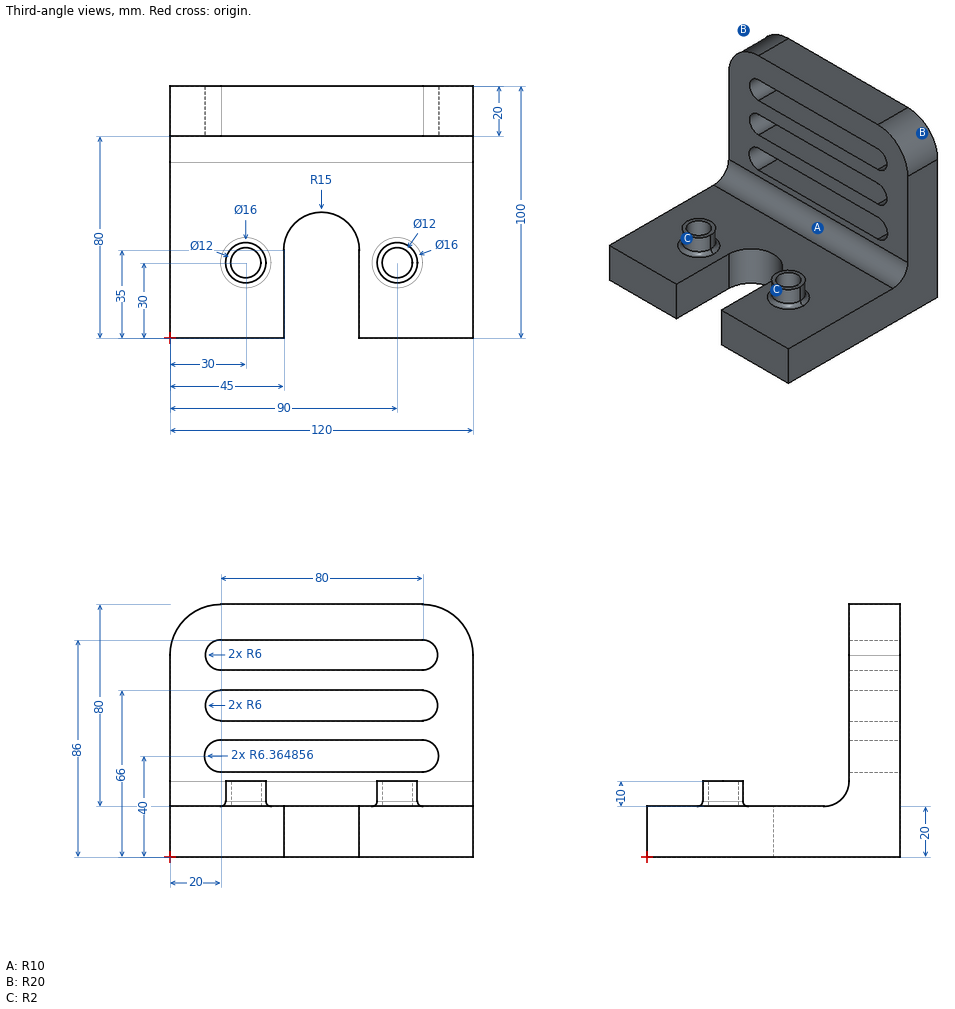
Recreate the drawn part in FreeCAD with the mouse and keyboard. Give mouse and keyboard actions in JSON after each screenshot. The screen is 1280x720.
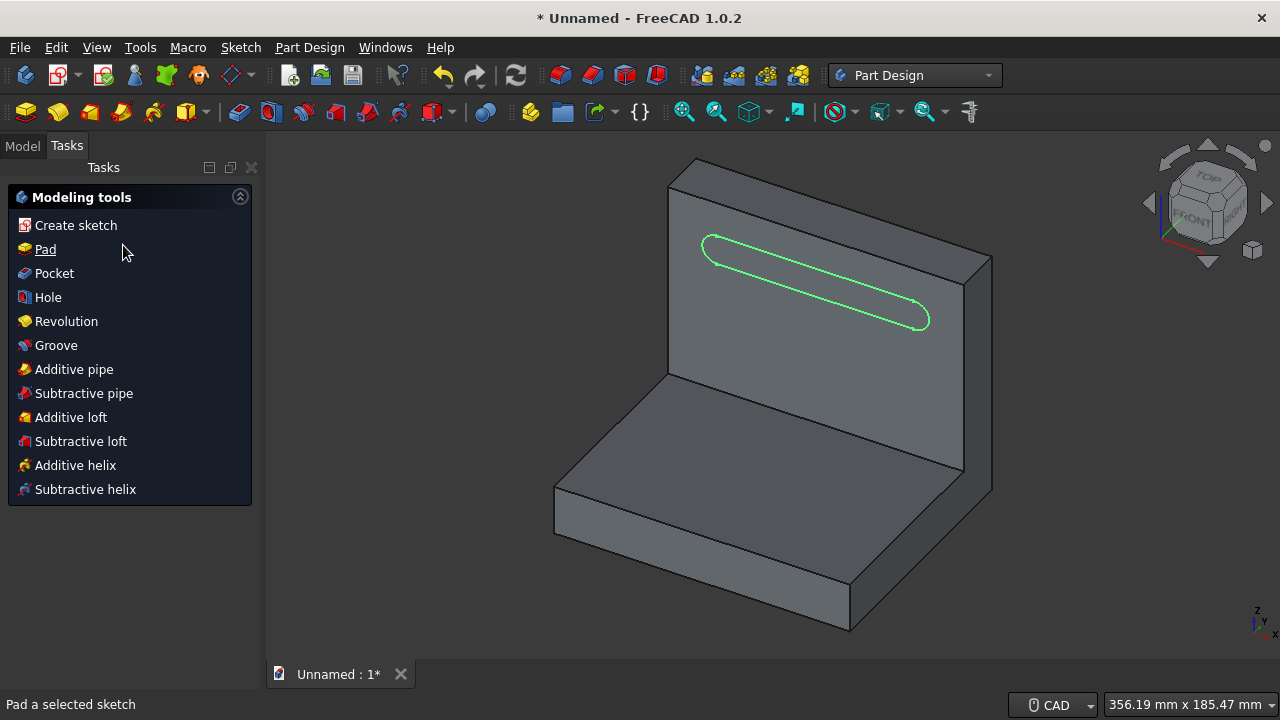
{"action": "left_click", "coordinate": [240, 112]}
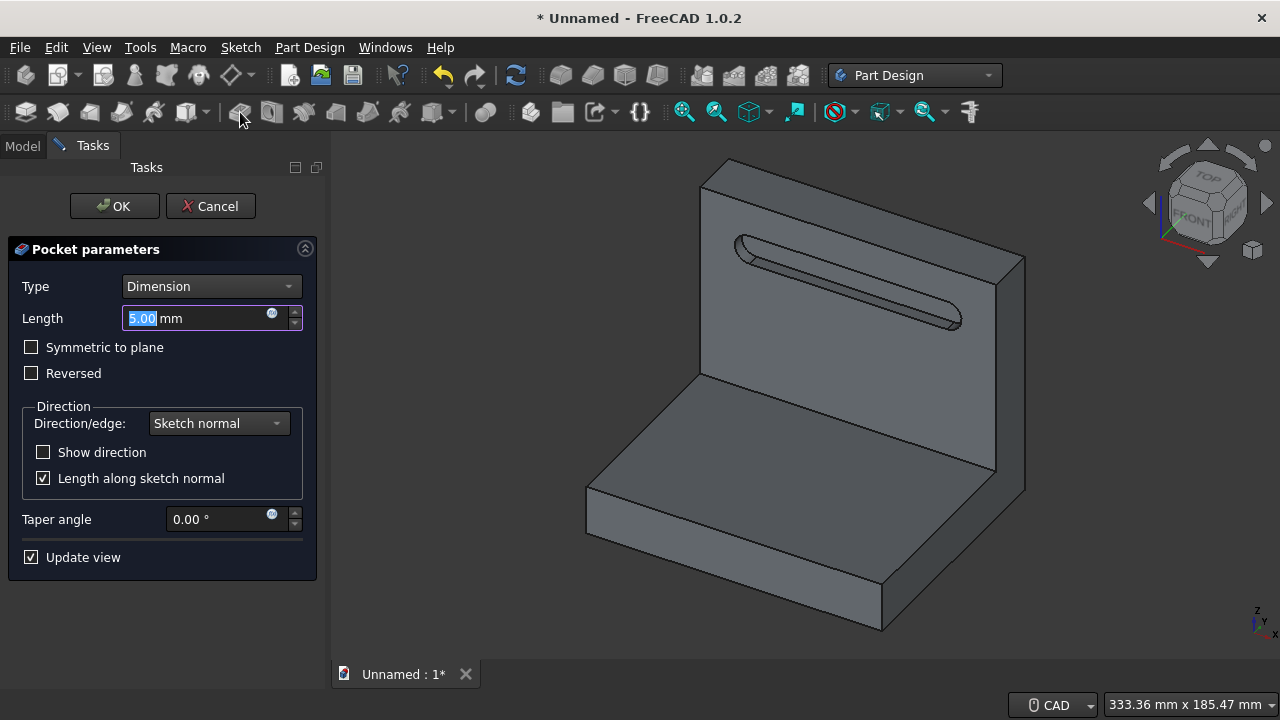
{"action": "left_click", "coordinate": [212, 286]}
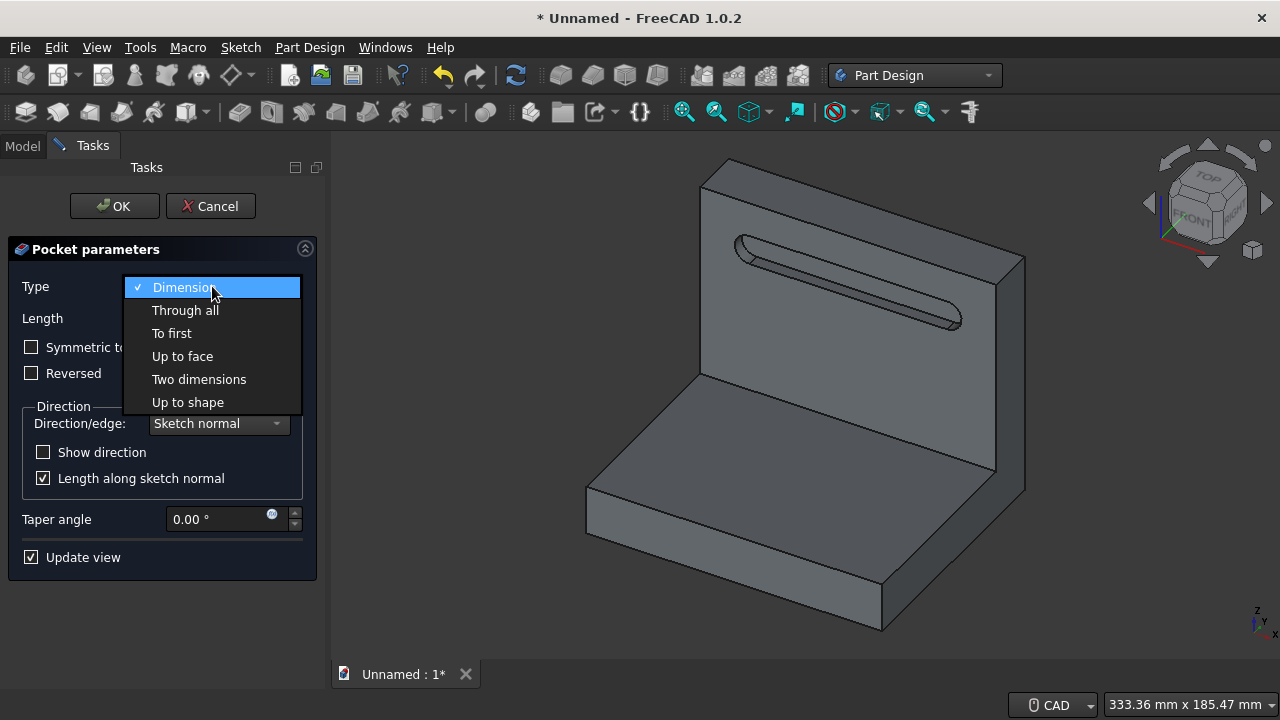
{"action": "left_click", "coordinate": [212, 310]}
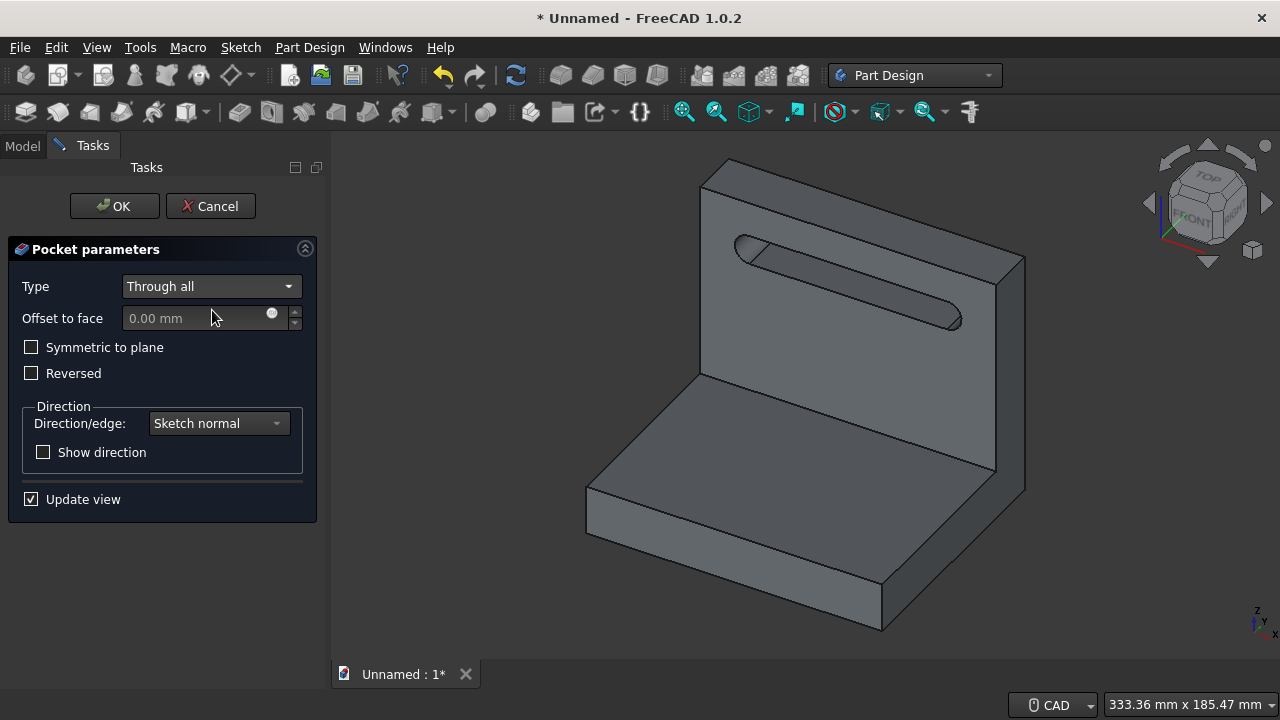
{"action": "left_click", "coordinate": [115, 206]}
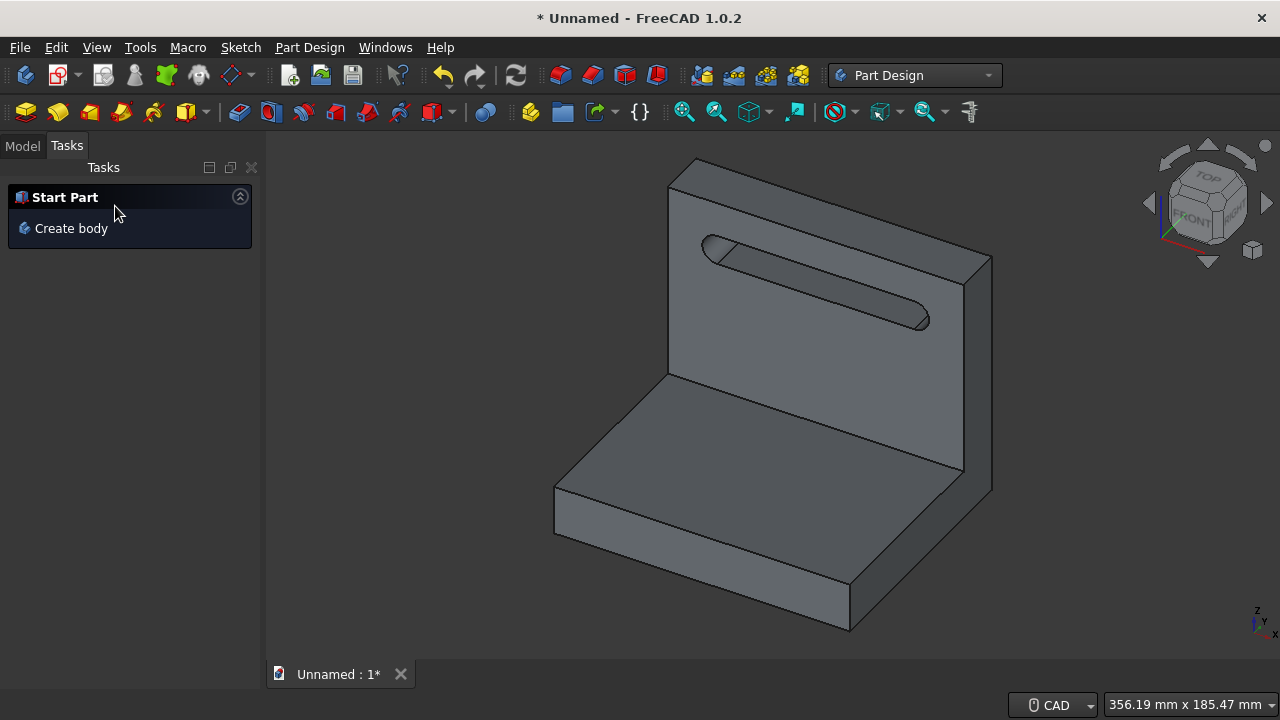
{"action": "left_click", "coordinate": [900, 383]}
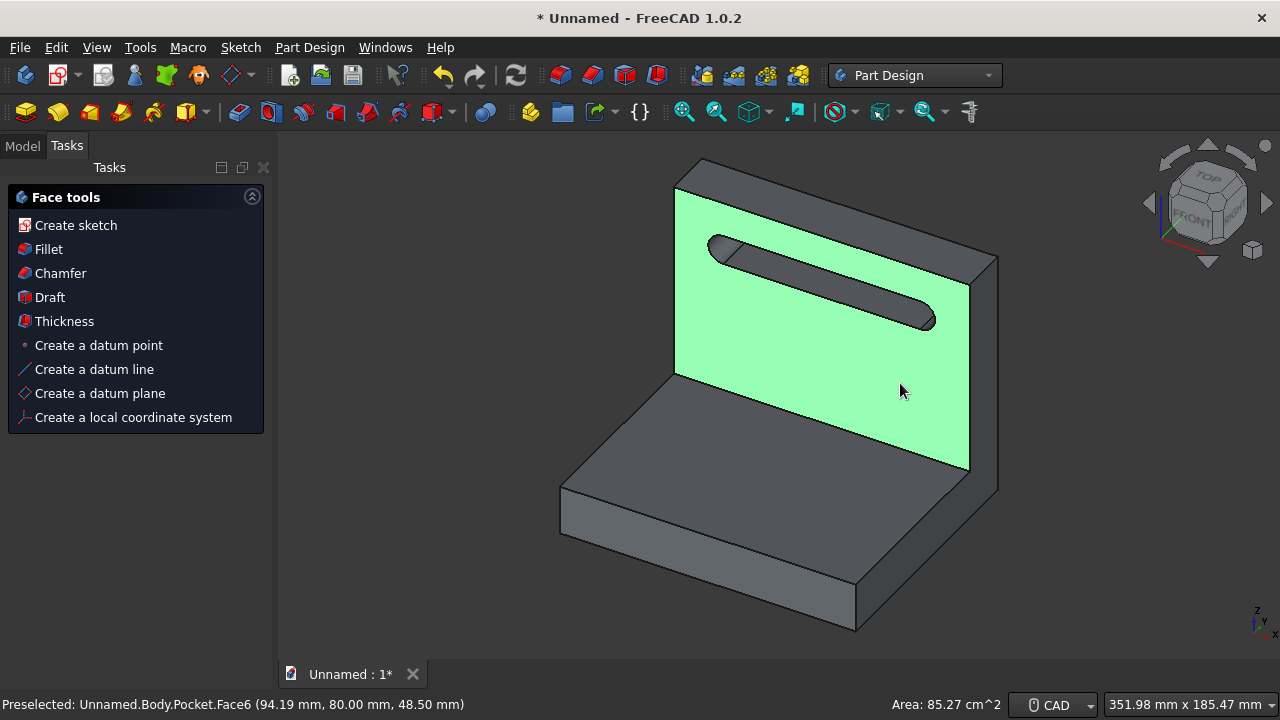
{"action": "left_click", "coordinate": [58, 76]}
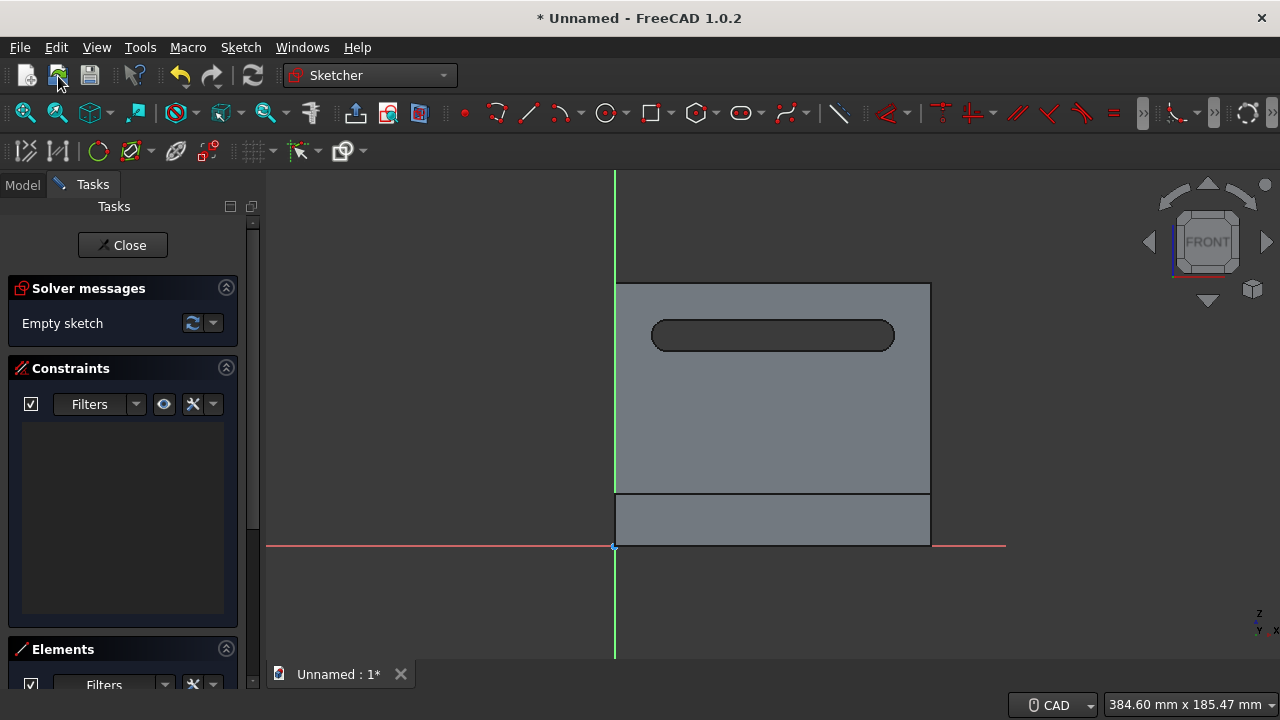
{"action": "key", "text": "q s"}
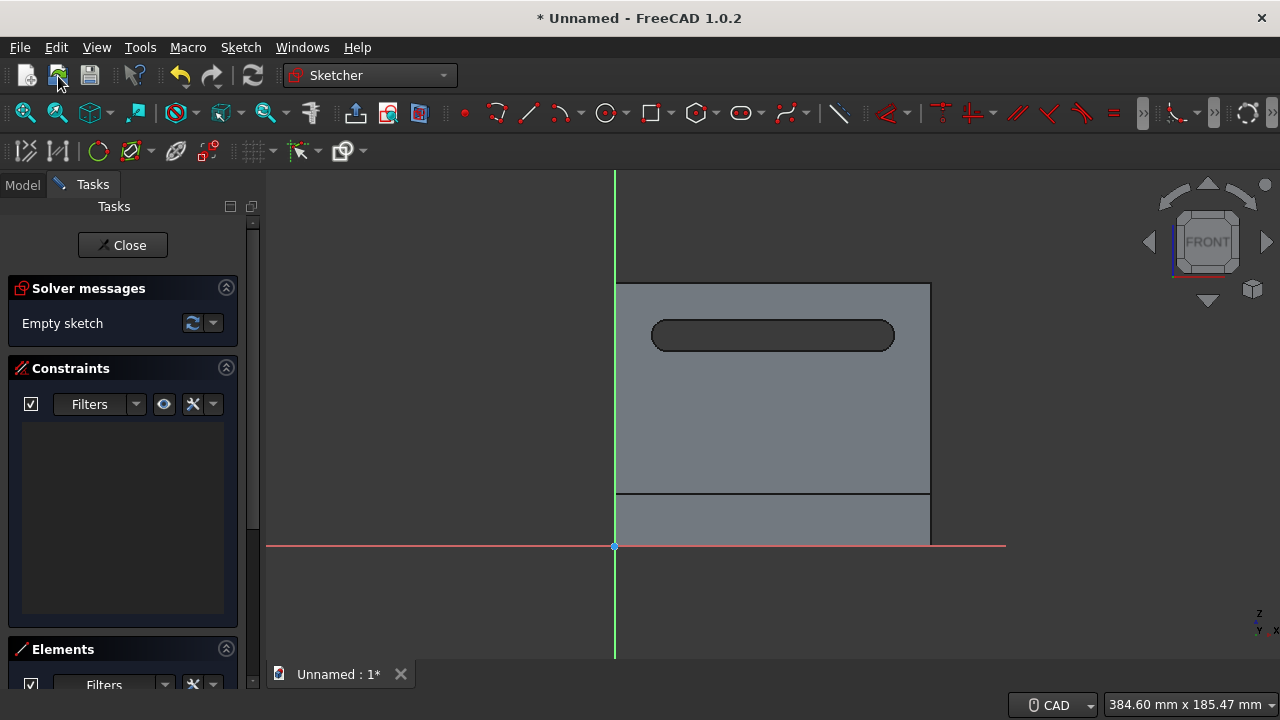
{"action": "scroll", "coordinate": [815, 514], "scroll_direction": "up", "scroll_amount": 3}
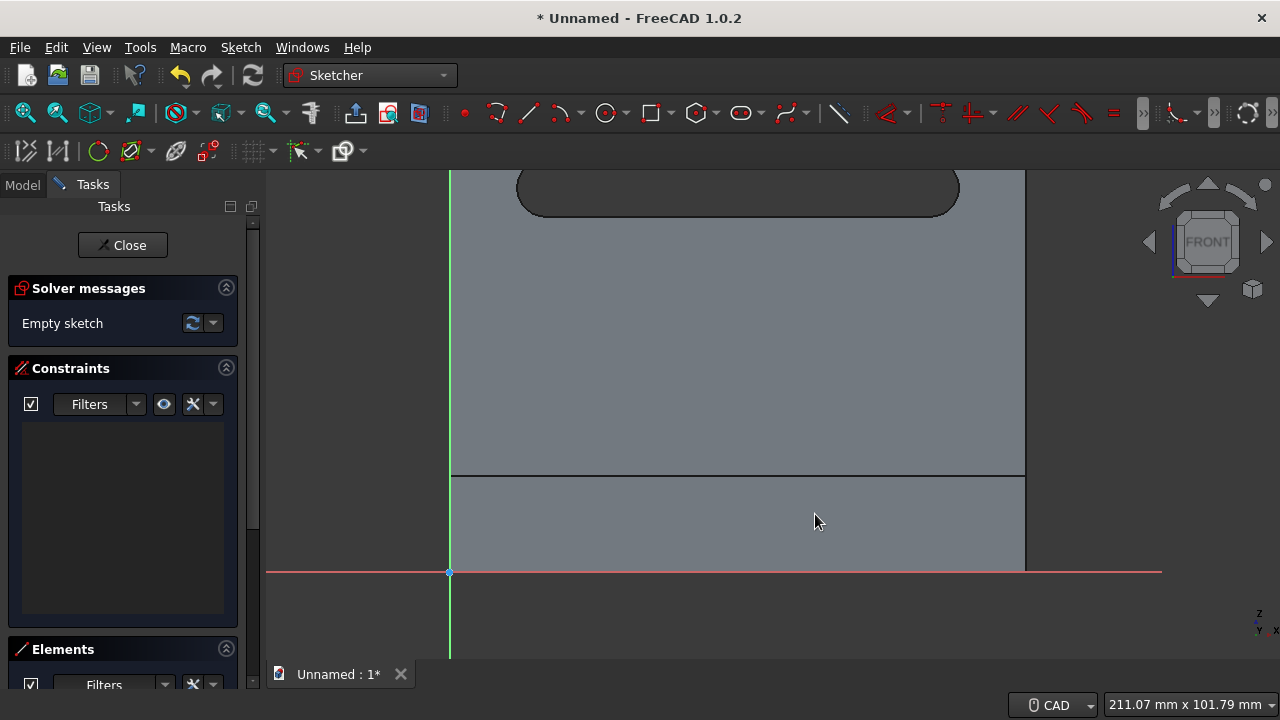
{"action": "key", "text": "g s"}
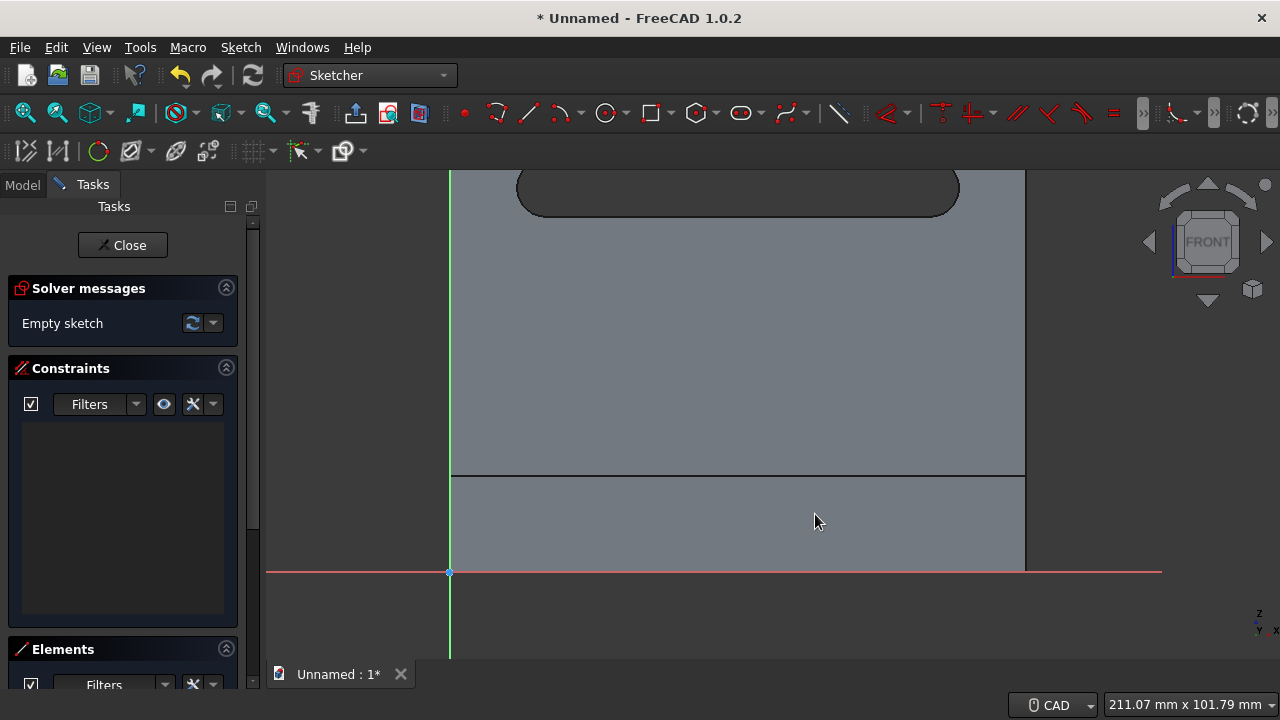
{"action": "left_click", "coordinate": [546, 284]}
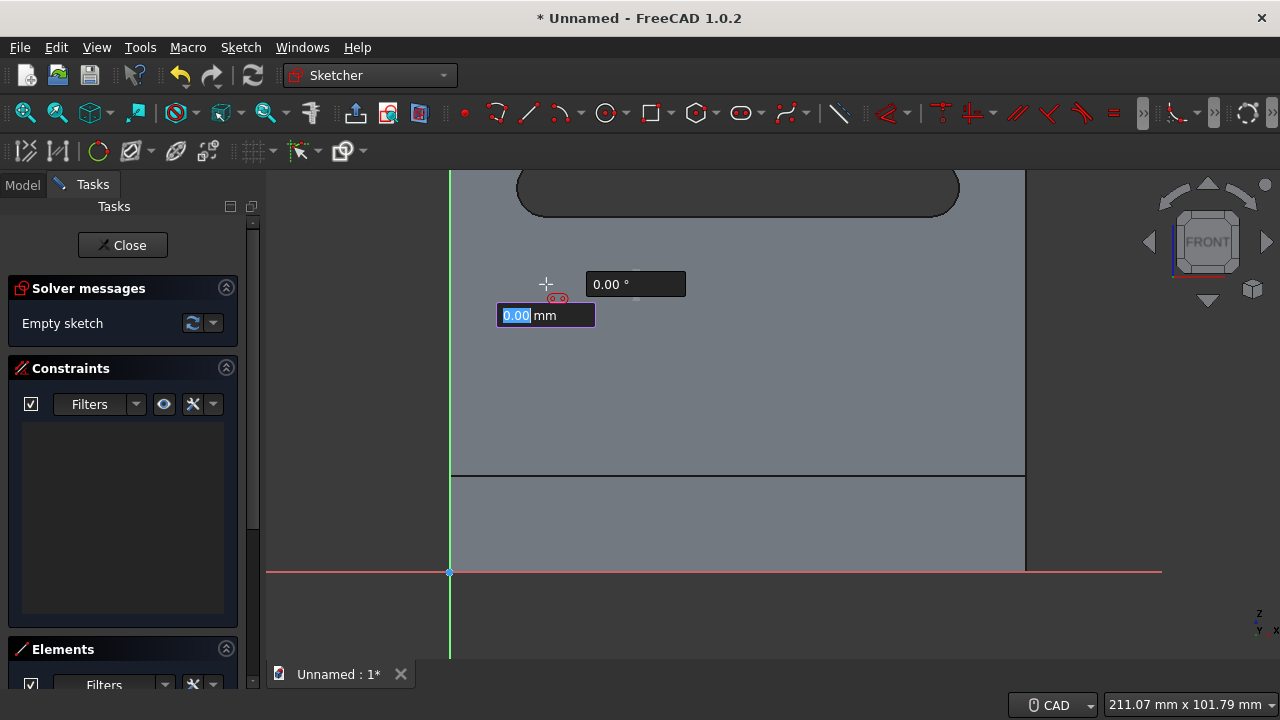
{"action": "left_click", "coordinate": [930, 284]}